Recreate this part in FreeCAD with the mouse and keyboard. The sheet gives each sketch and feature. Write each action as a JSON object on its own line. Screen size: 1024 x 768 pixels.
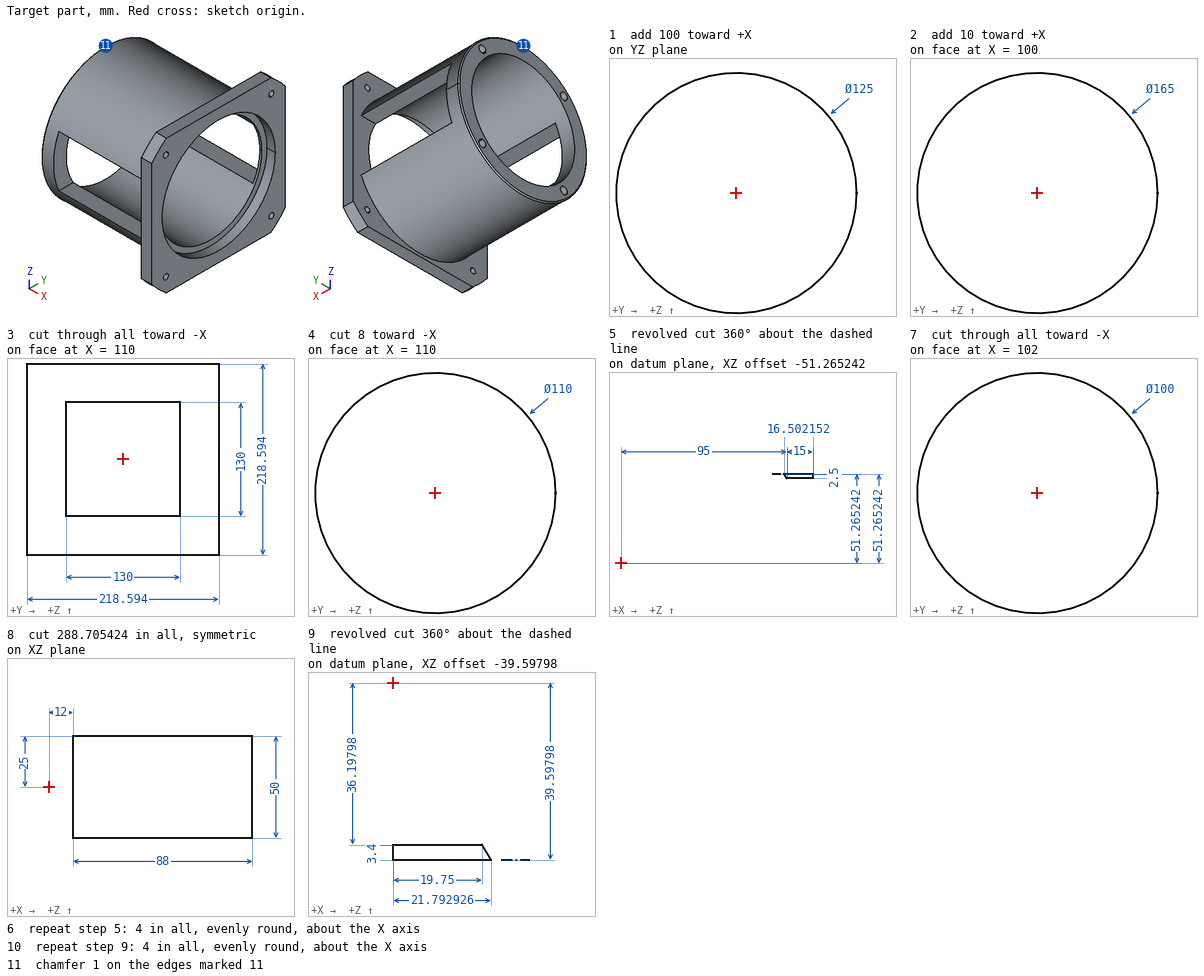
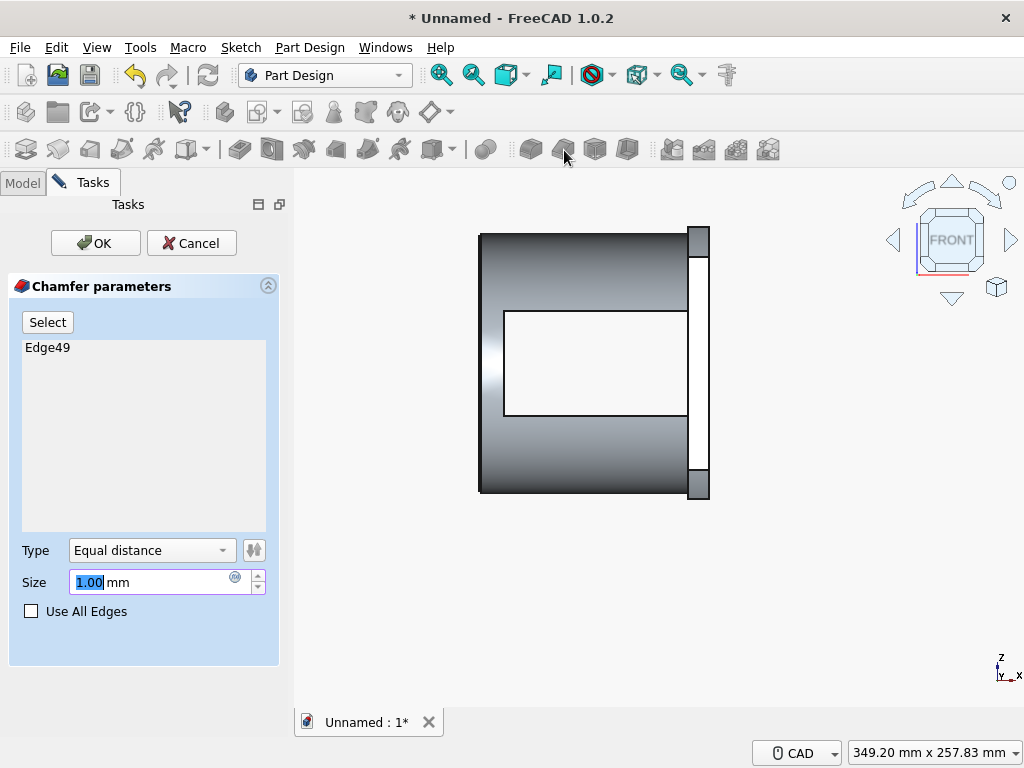
{"action": "type", "text": "1"}
{"action": "key", "text": "Tab"}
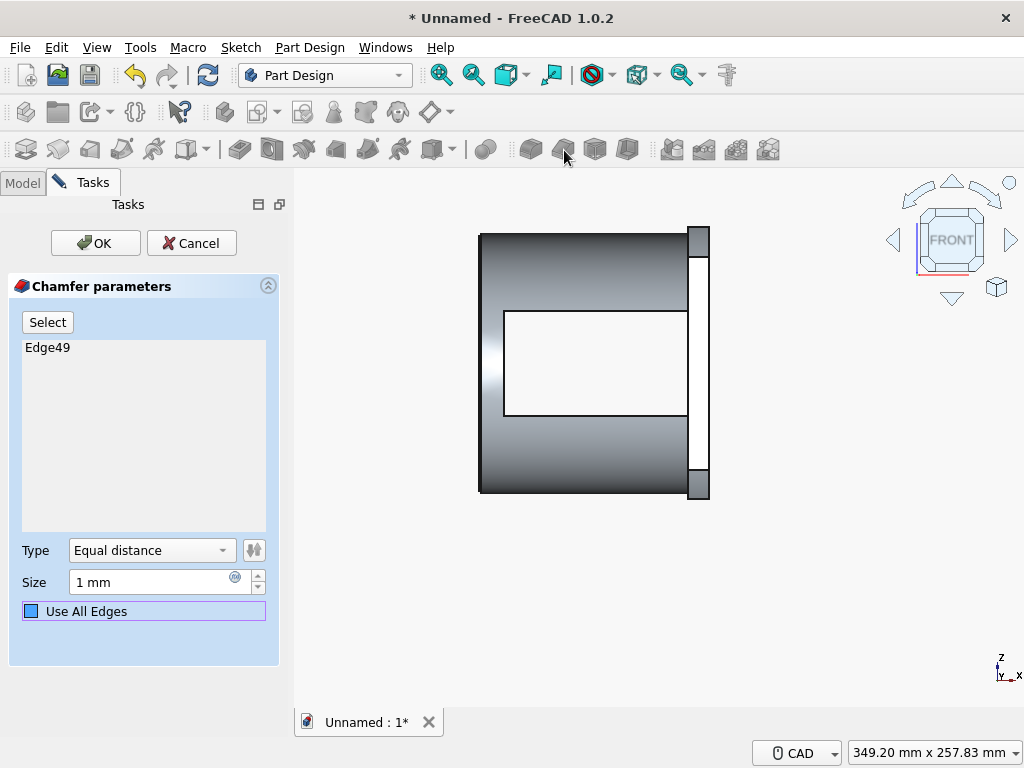
{"action": "left_click", "coordinate": [96, 243]}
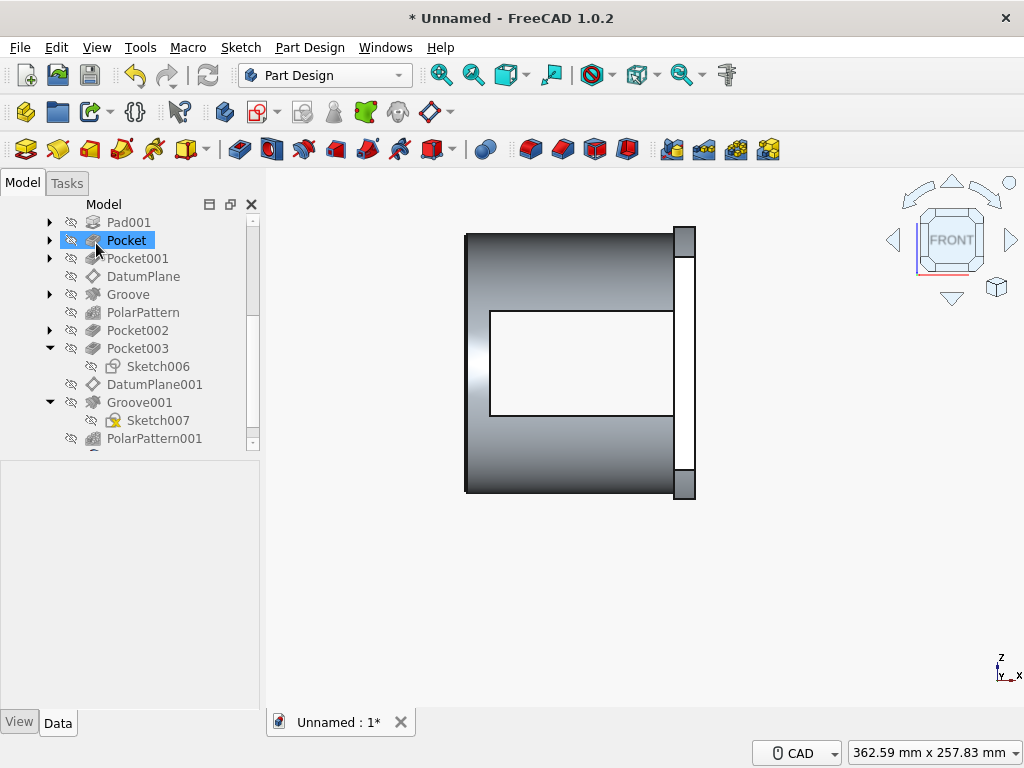
{"action": "key", "text": "0"}